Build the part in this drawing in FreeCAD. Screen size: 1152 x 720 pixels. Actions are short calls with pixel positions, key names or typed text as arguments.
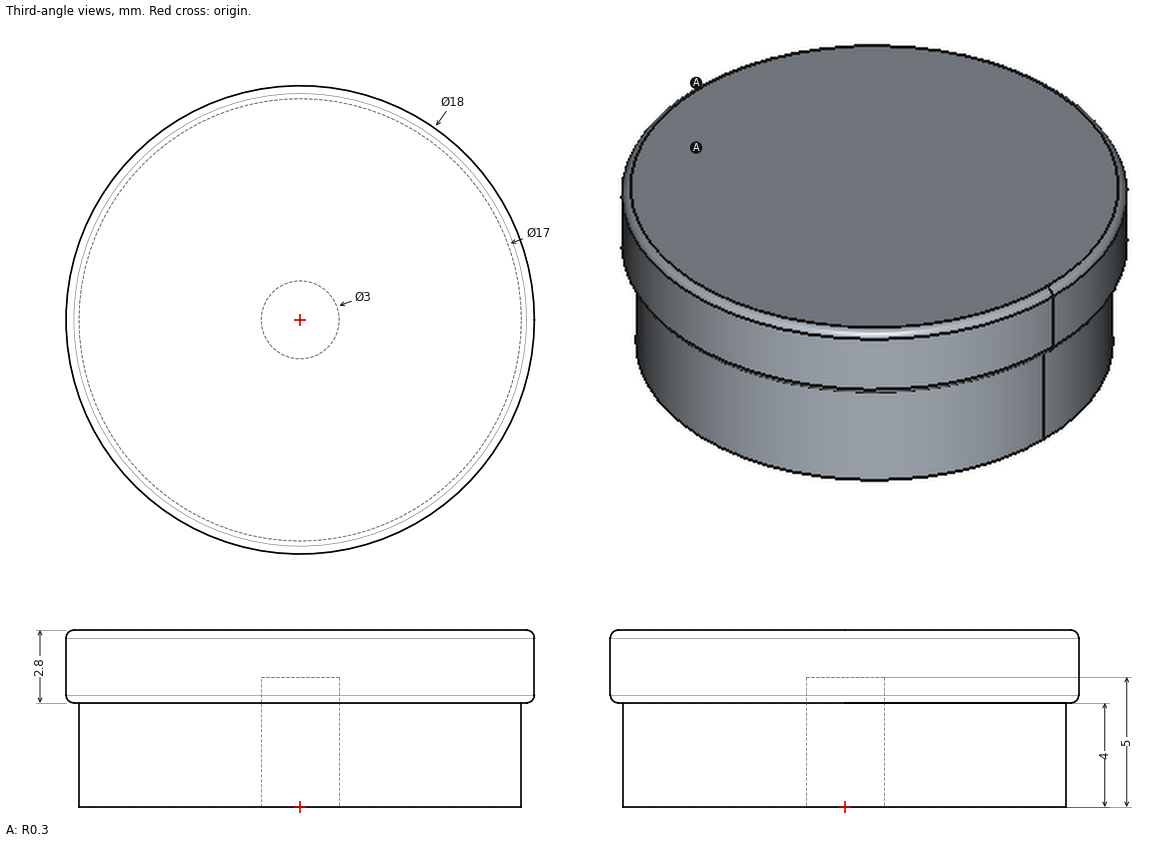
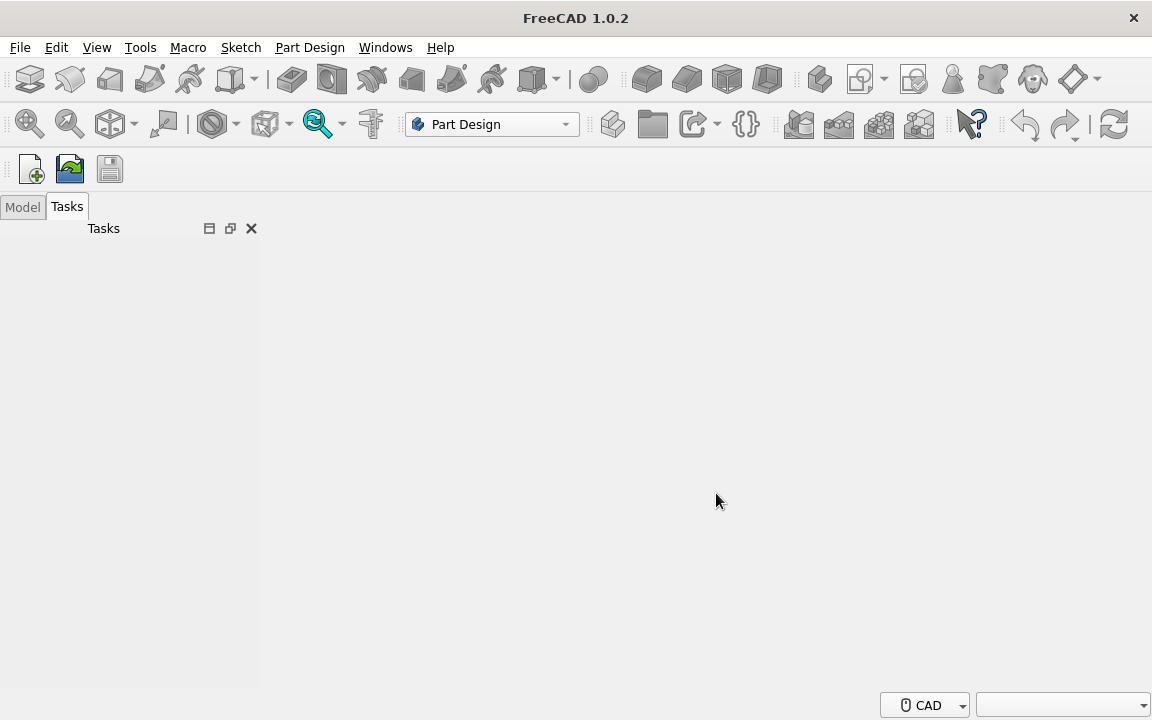
click(30, 170)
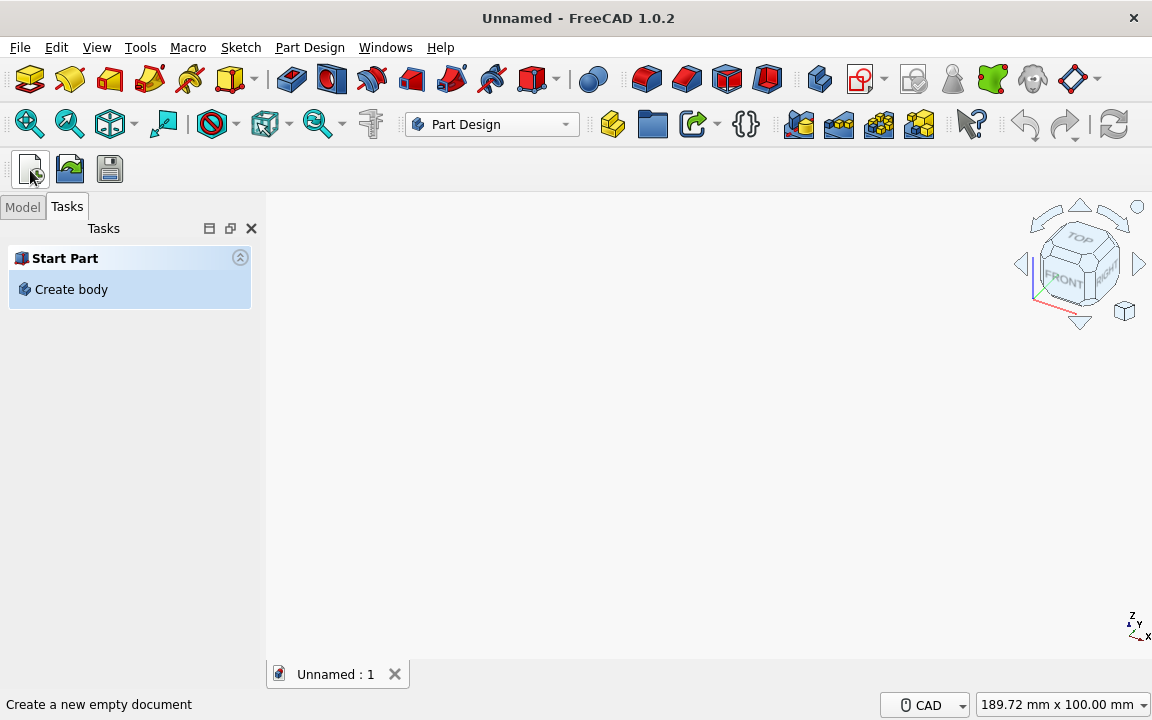
click(860, 80)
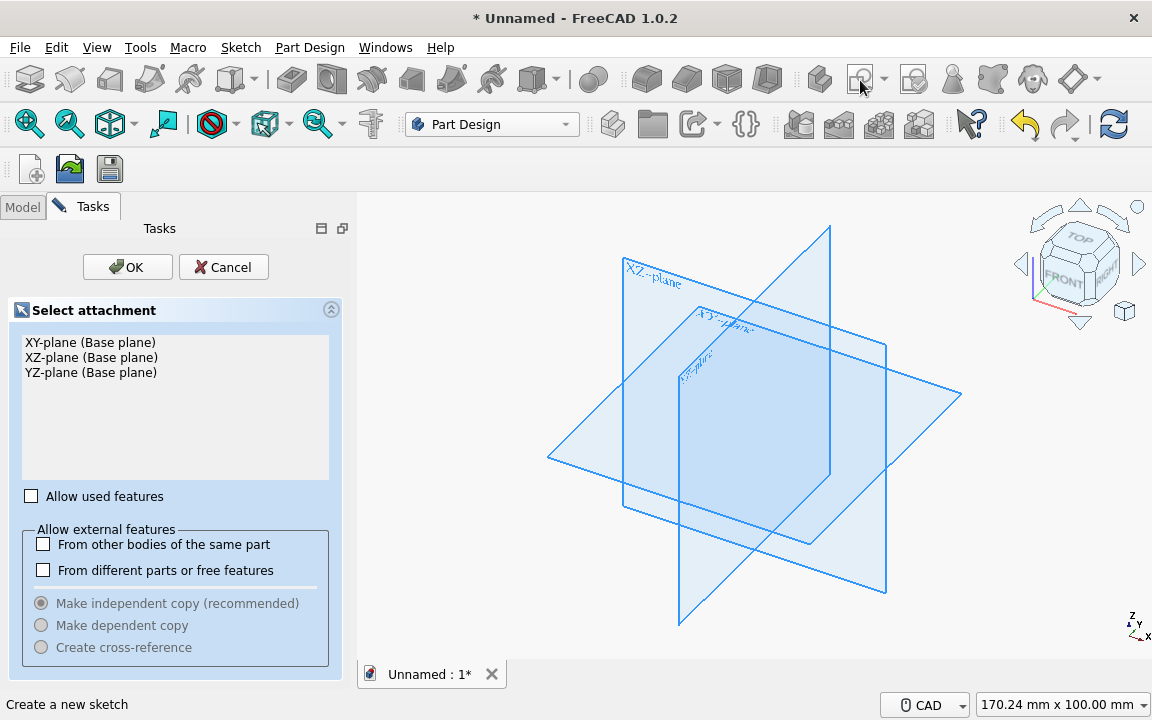
click(82, 342)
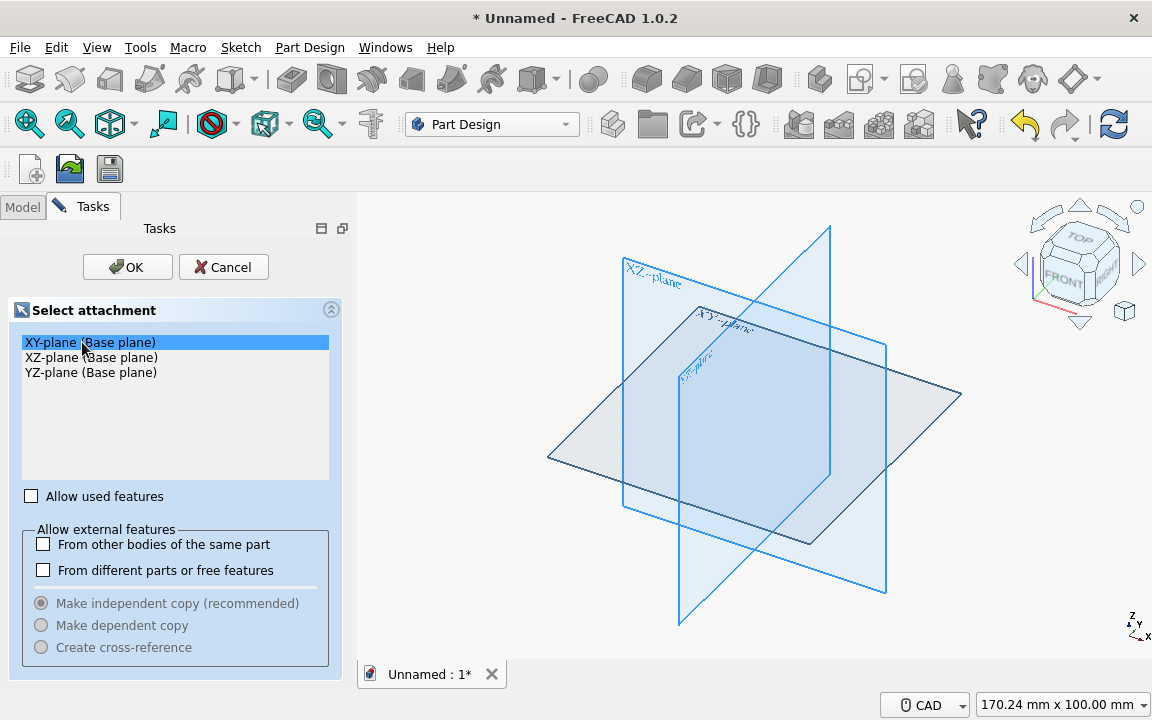
click(128, 267)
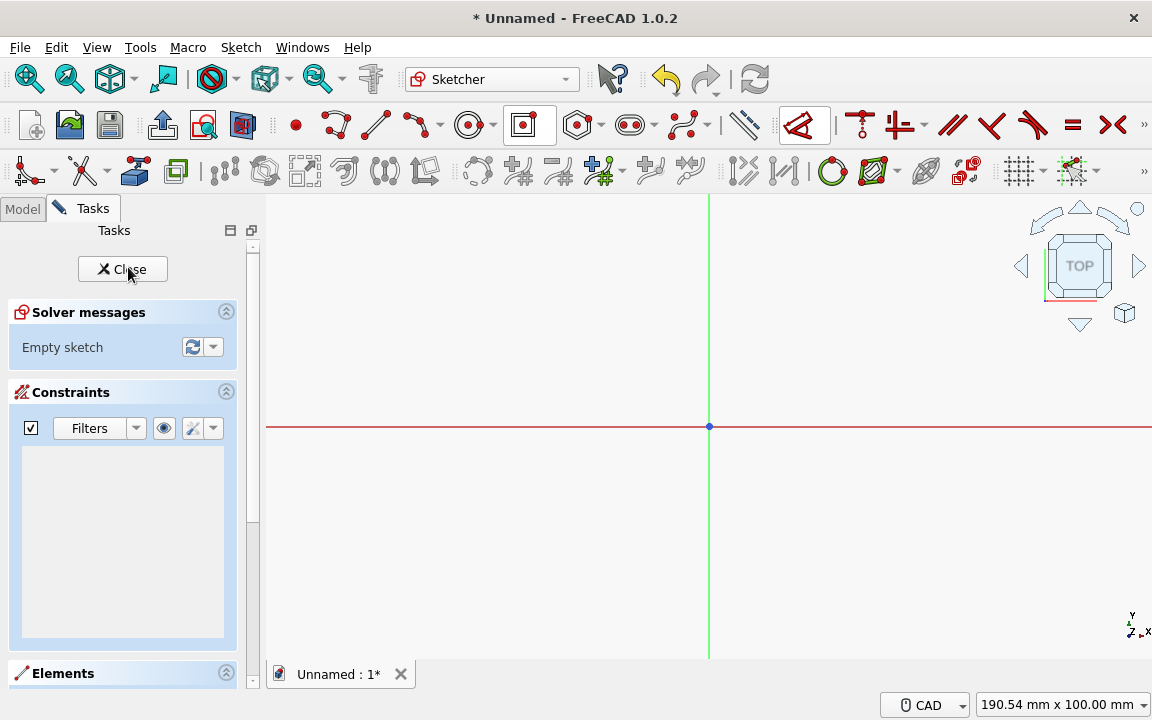
scroll(739, 427, up, 6)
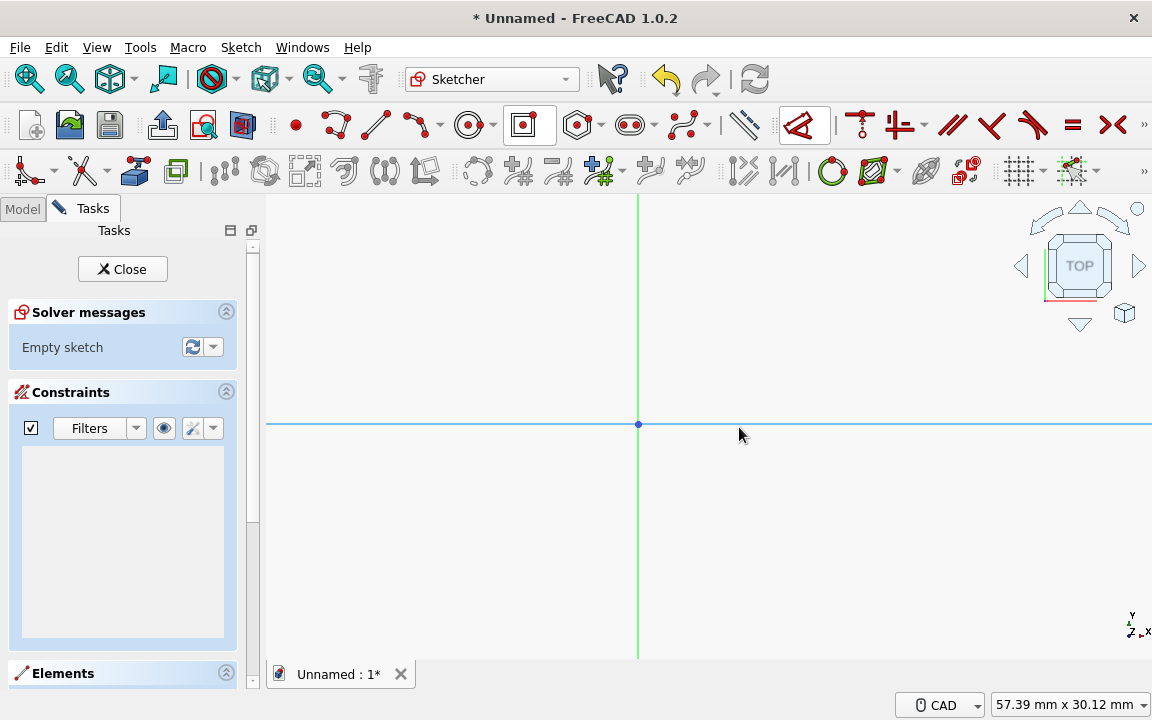
key(g)
key(c)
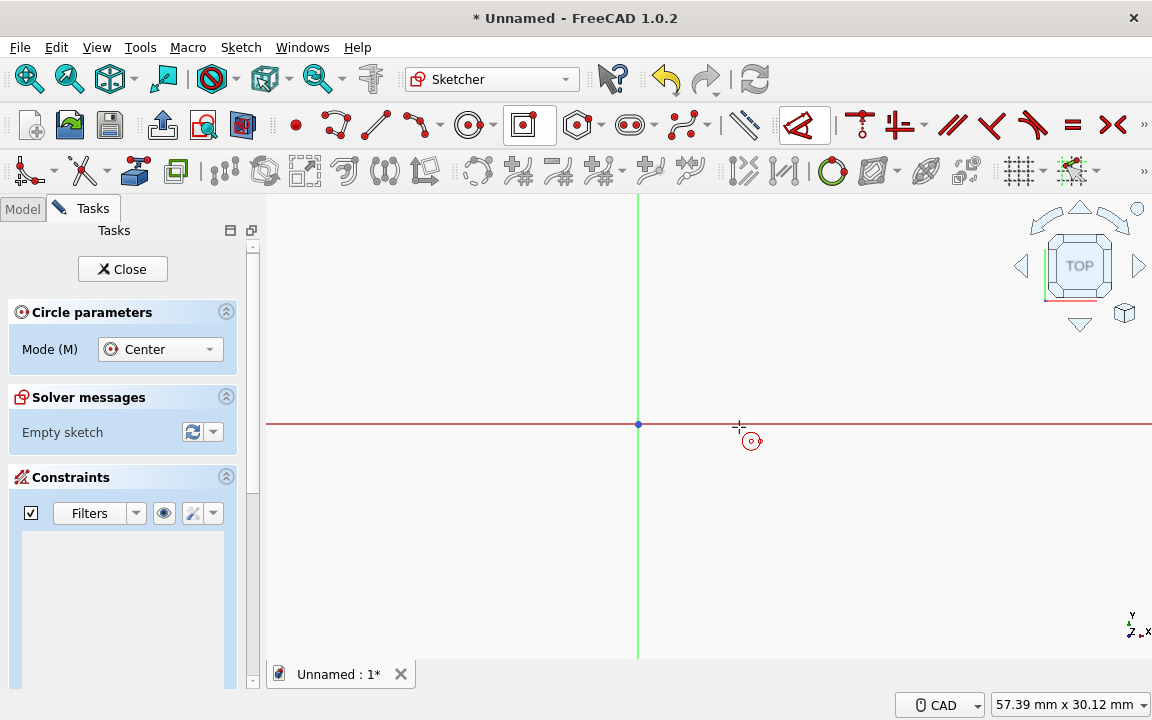
click(638, 424)
move(731, 331)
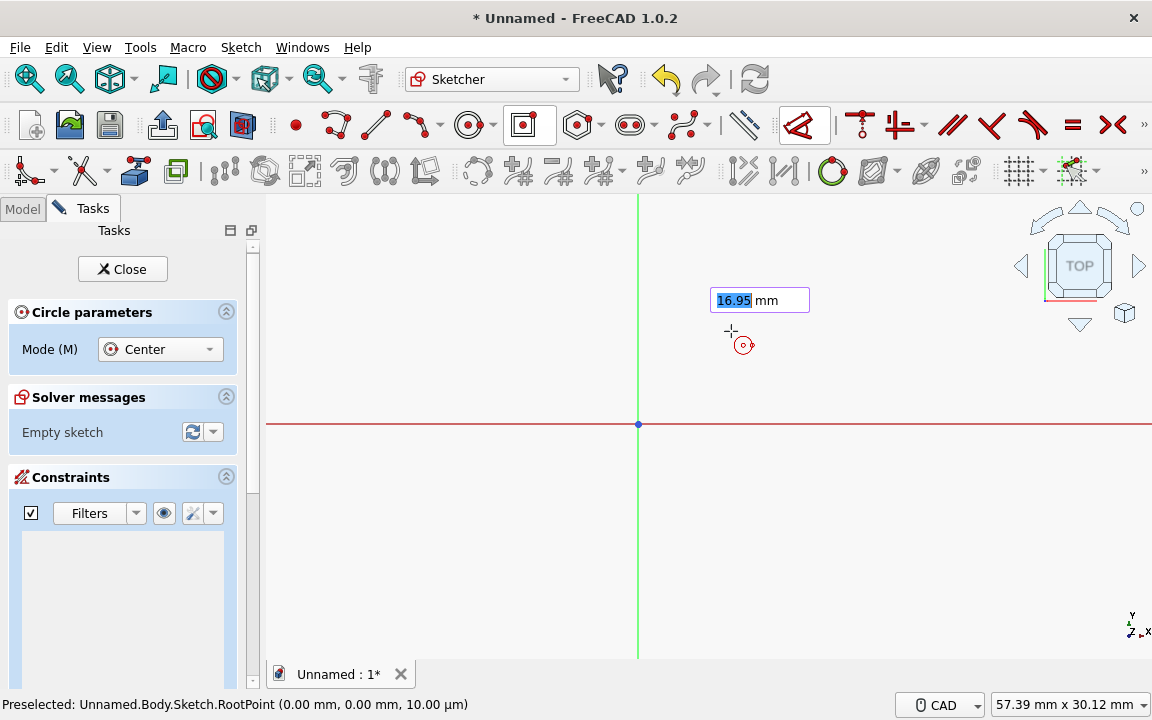
text(17)
key(Return)
key(Escape)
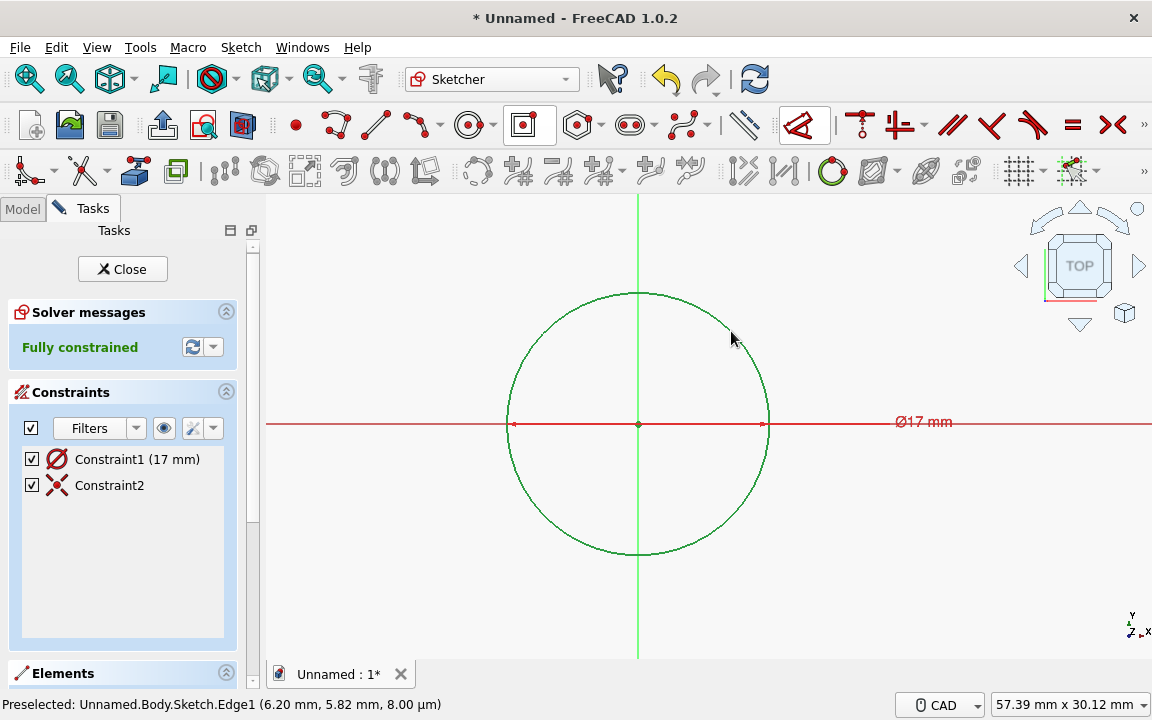
click(123, 269)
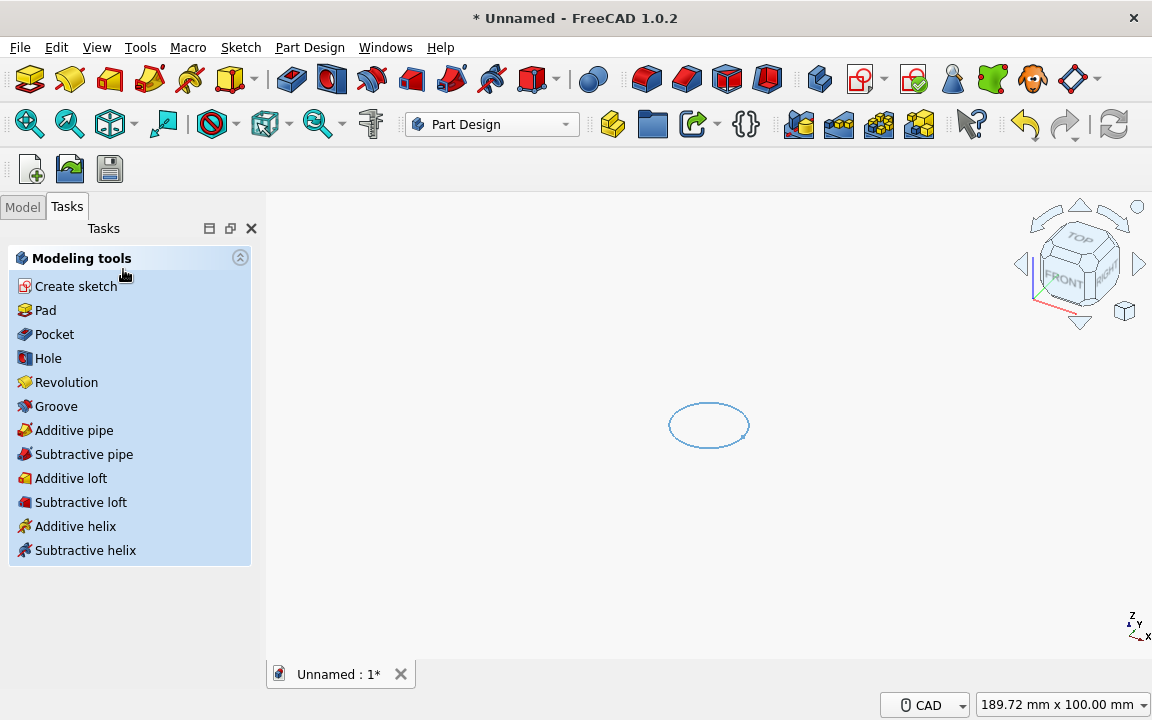
click(30, 80)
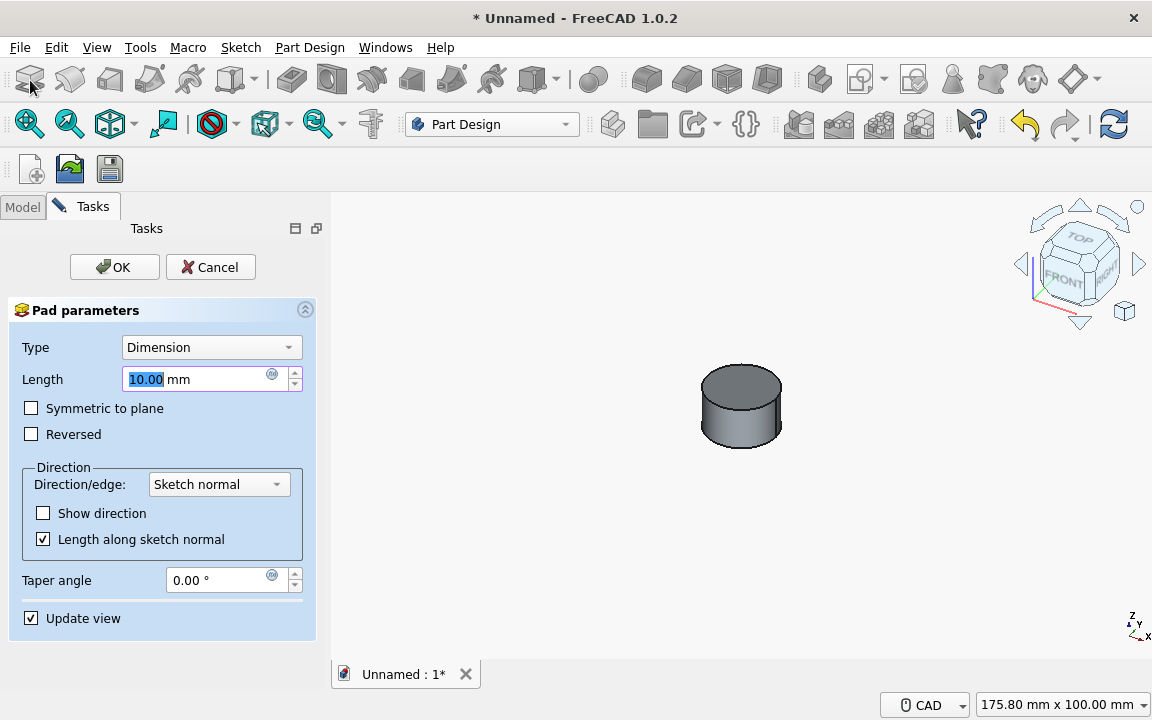
text(4)
key(Tab)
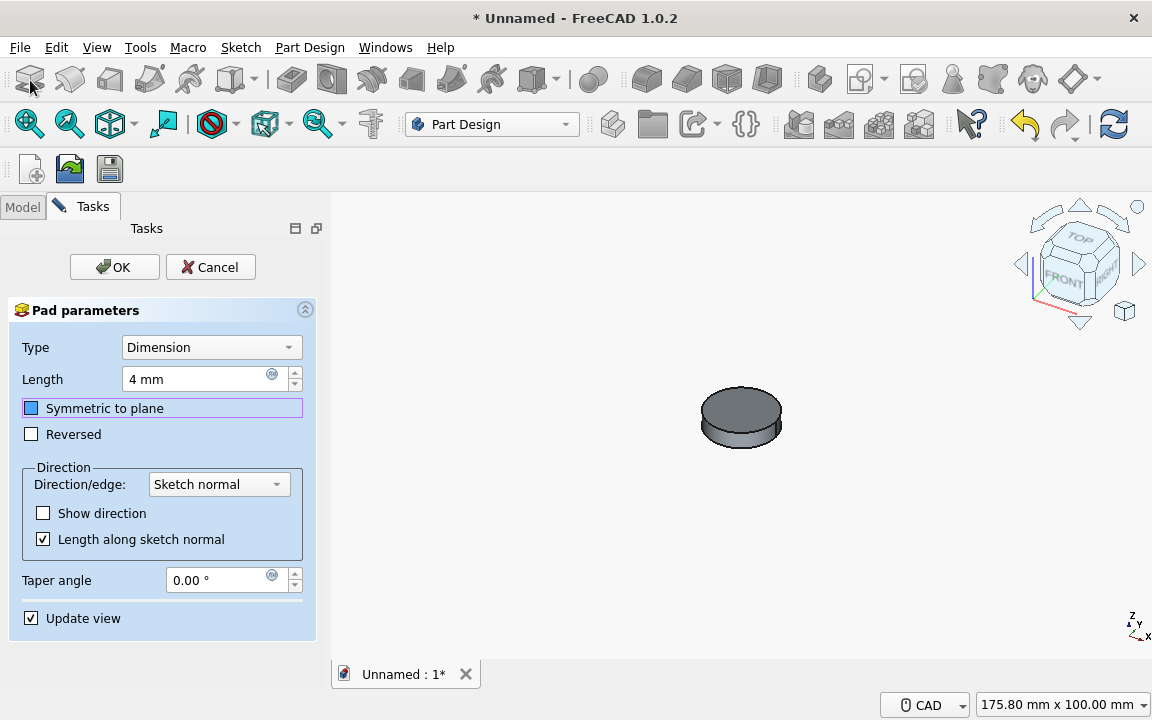
click(115, 267)